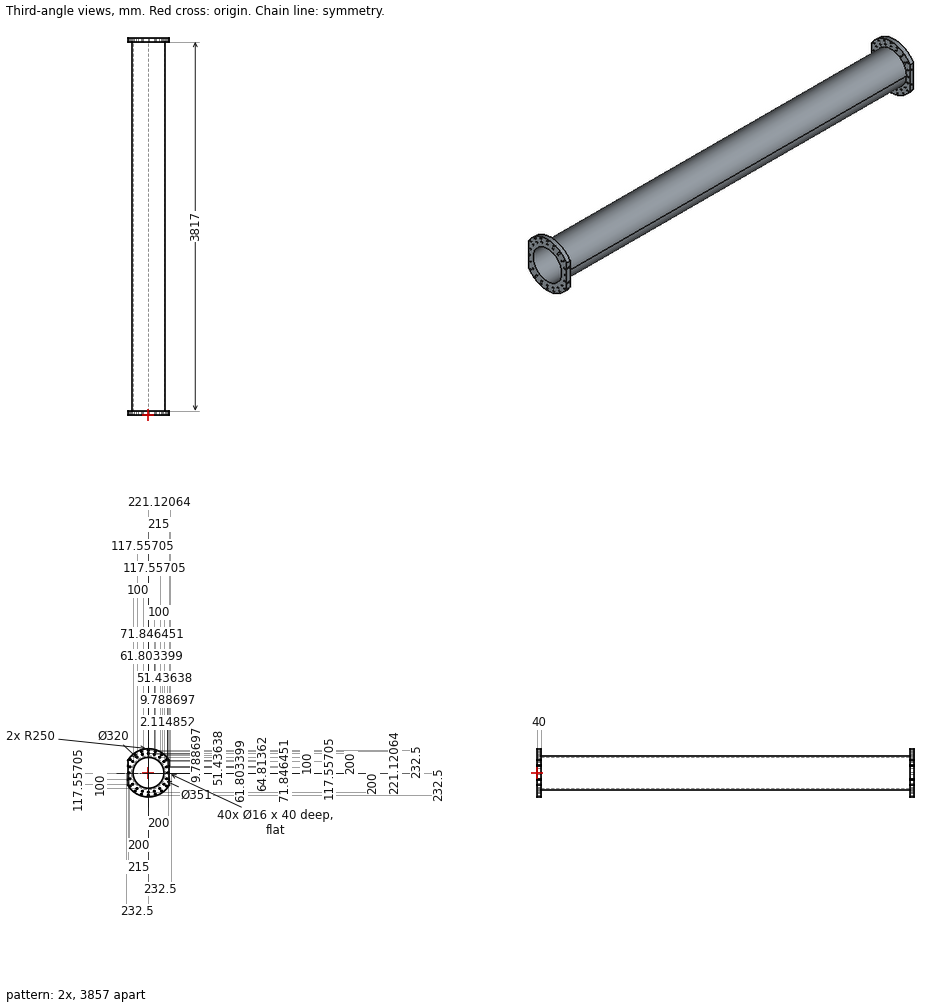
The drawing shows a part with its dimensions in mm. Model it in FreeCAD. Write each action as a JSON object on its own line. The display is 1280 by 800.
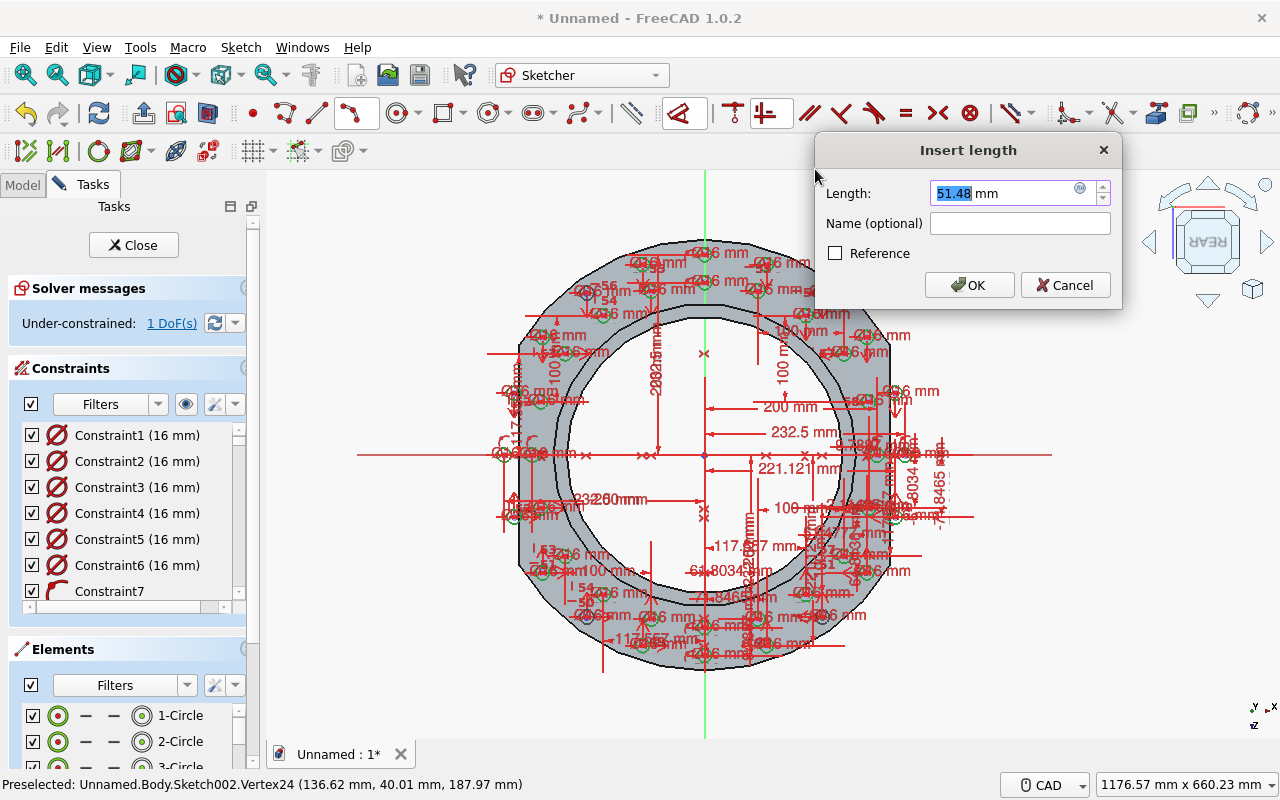
{"action": "type", "text": "51.43638"}
{"action": "key", "text": "Return"}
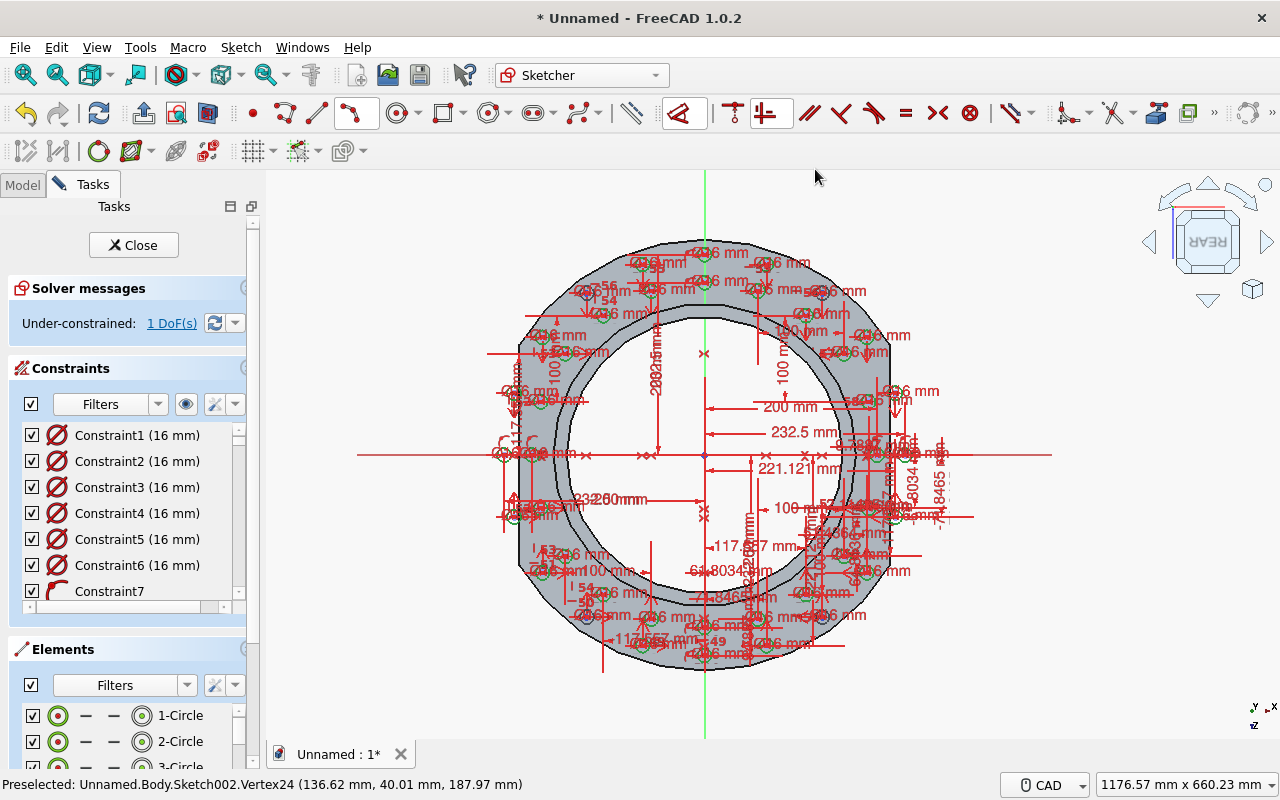
{"action": "left_click", "coordinate": [867, 573]}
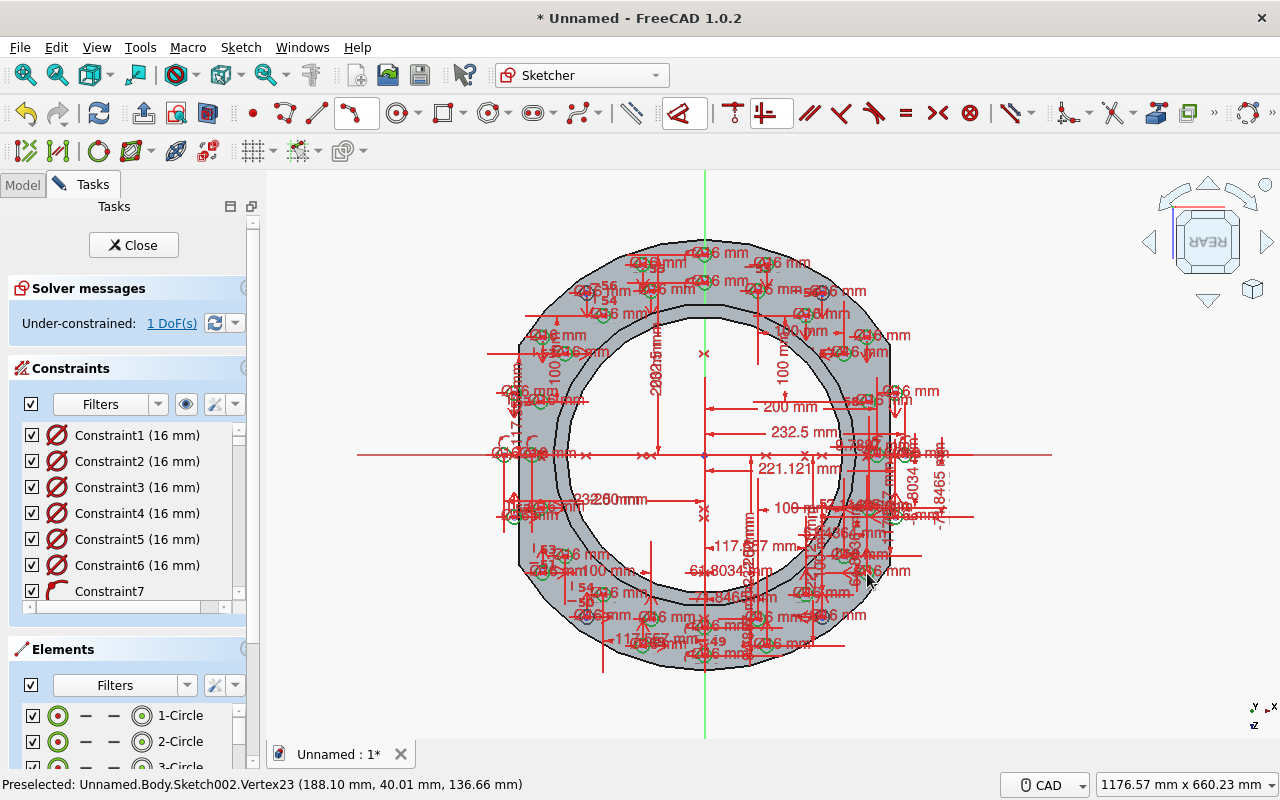
{"action": "left_click", "coordinate": [822, 617]}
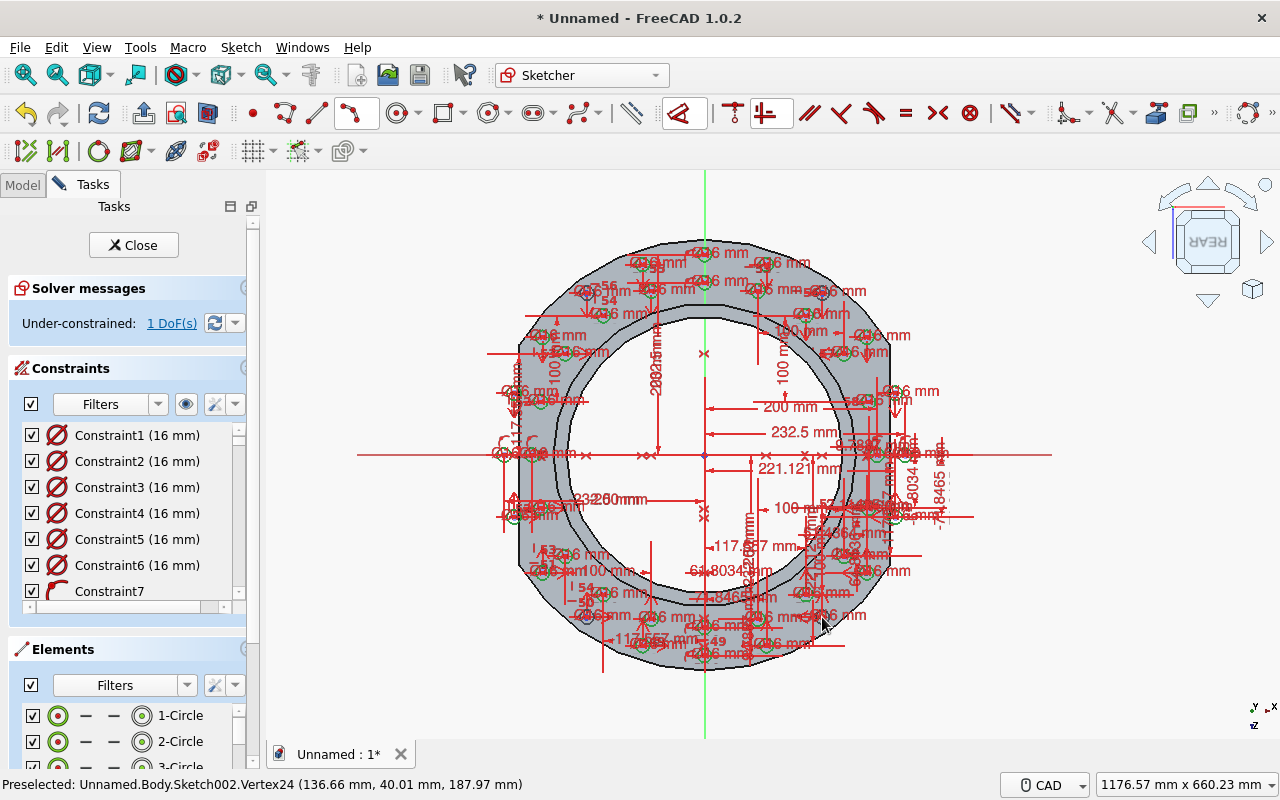
{"action": "left_click", "coordinate": [702, 114]}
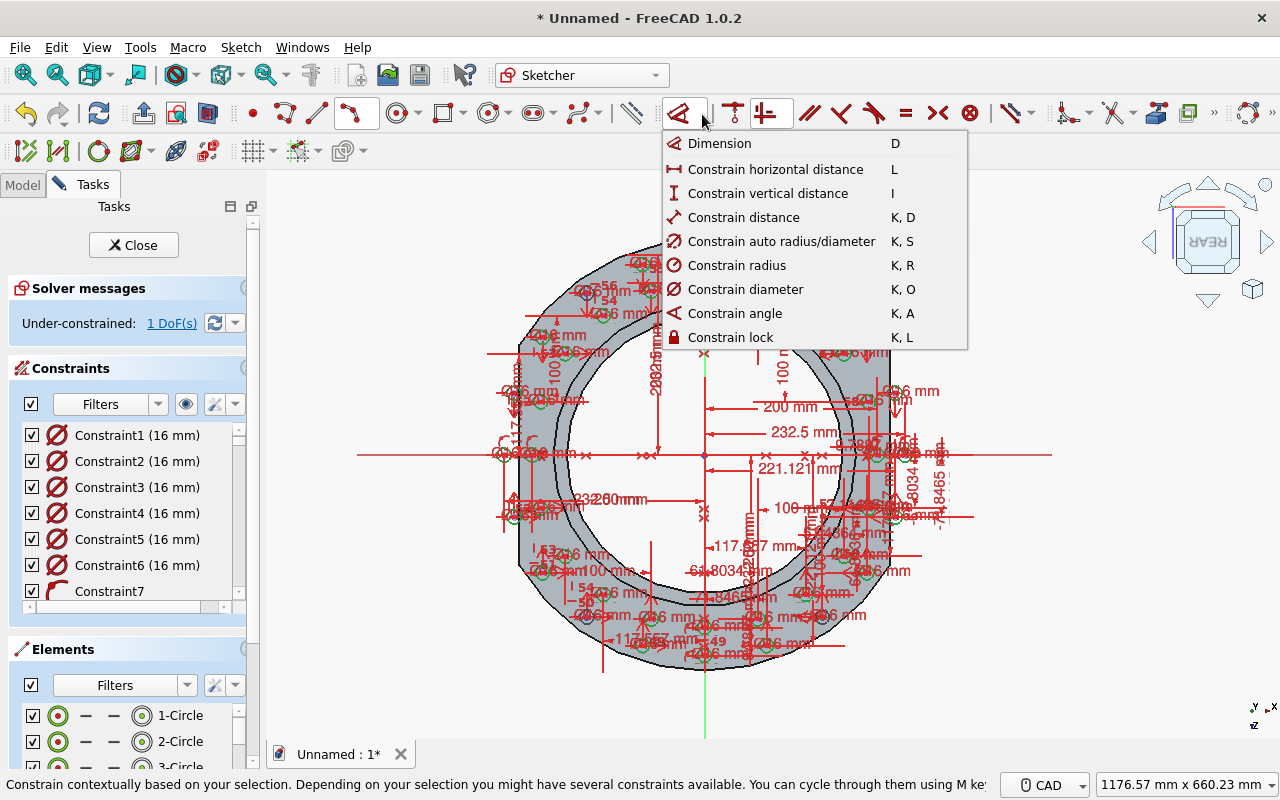
{"action": "left_click", "coordinate": [815, 193]}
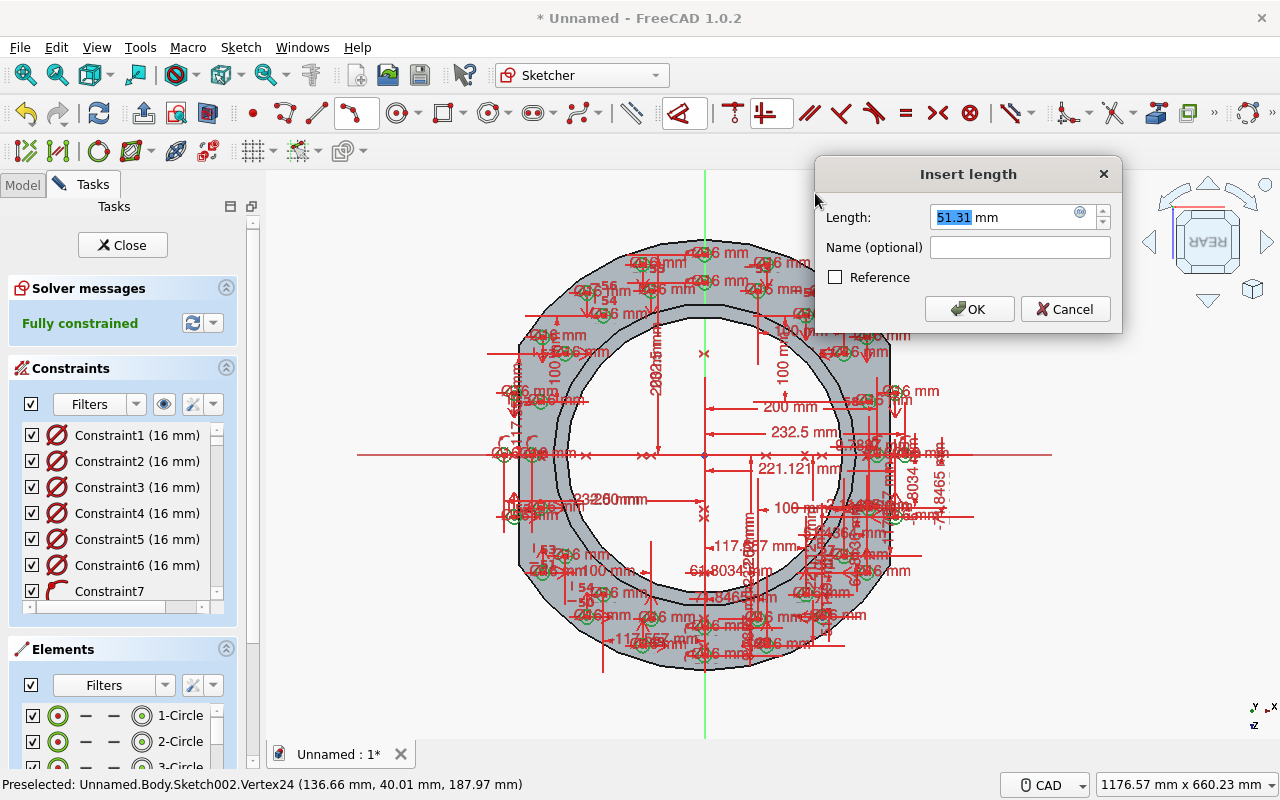
{"action": "type", "text": "51.43638"}
{"action": "key", "text": "Return"}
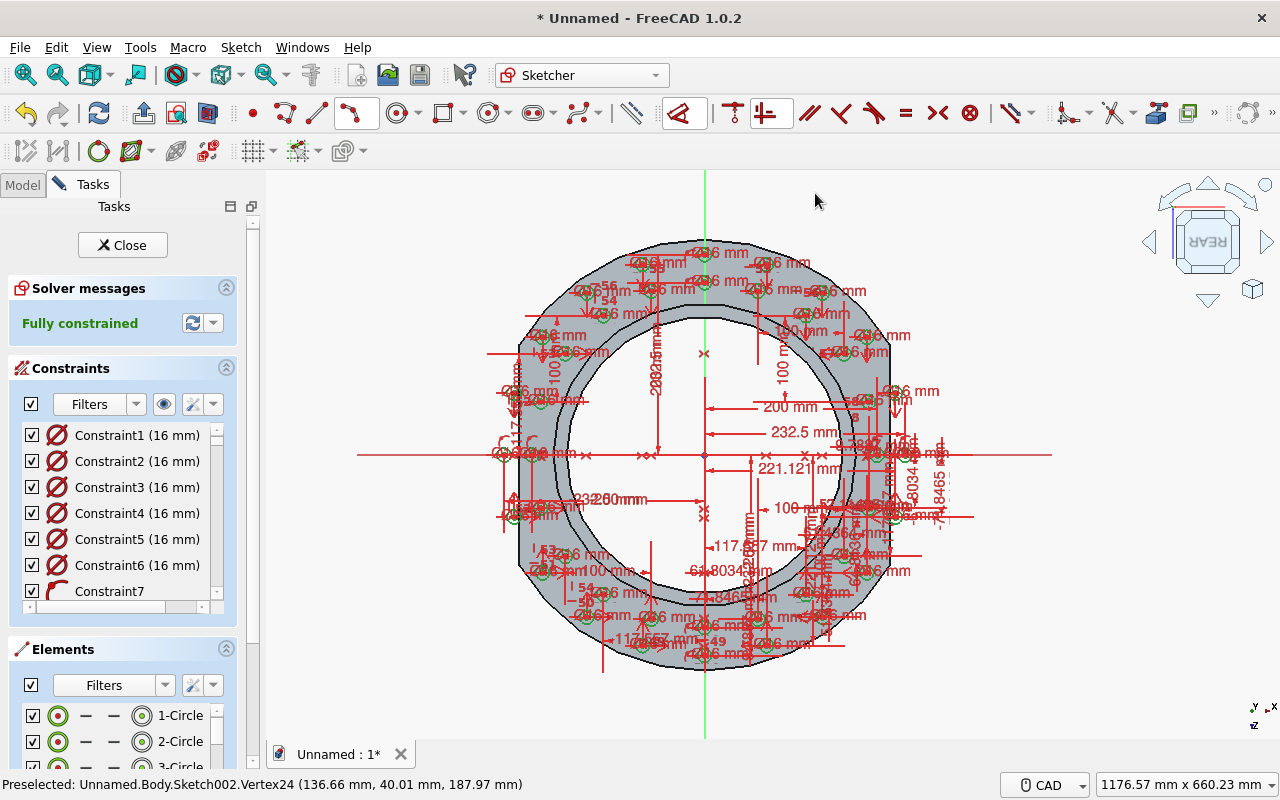
{"action": "left_click", "coordinate": [123, 245]}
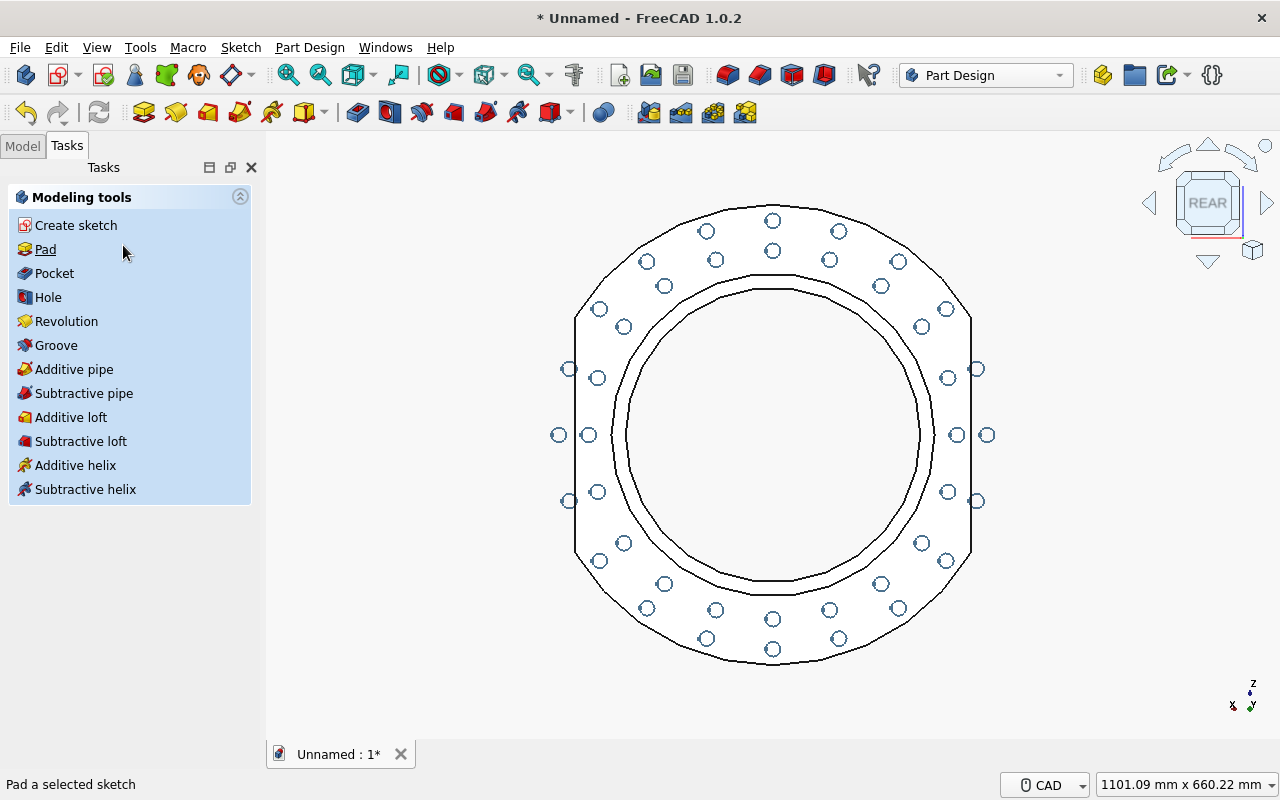
{"action": "left_click", "coordinate": [390, 112]}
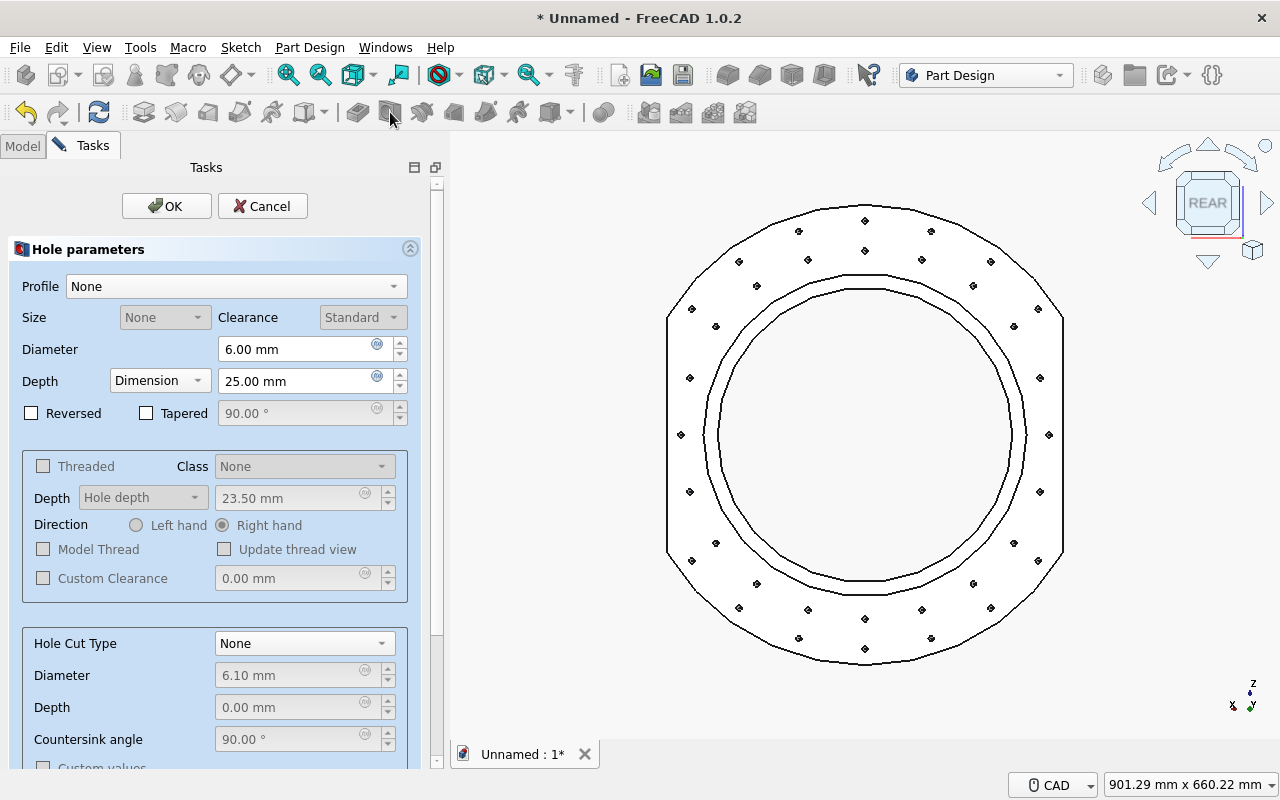
{"action": "triple_click", "coordinate": [305, 349]}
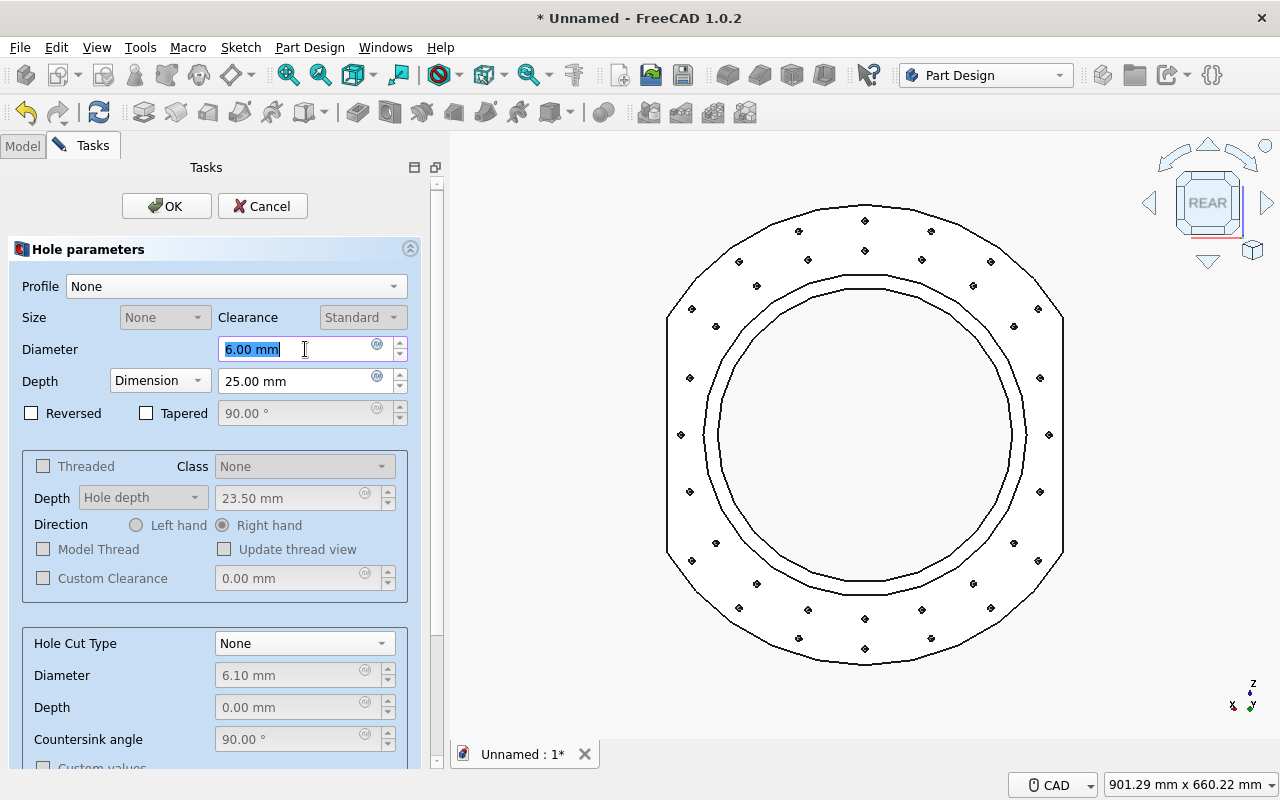
{"action": "type", "text": "16"}
{"action": "key", "text": "Tab"}